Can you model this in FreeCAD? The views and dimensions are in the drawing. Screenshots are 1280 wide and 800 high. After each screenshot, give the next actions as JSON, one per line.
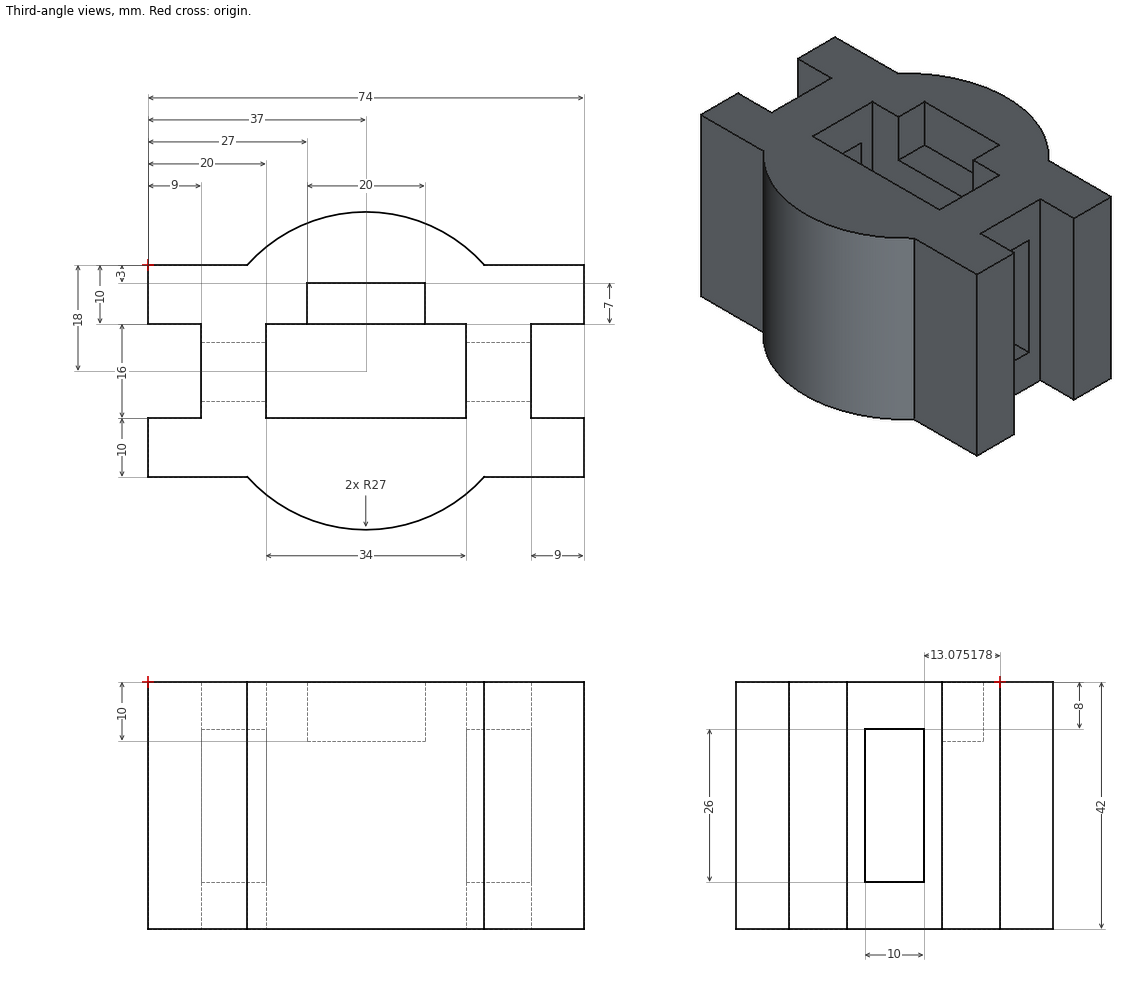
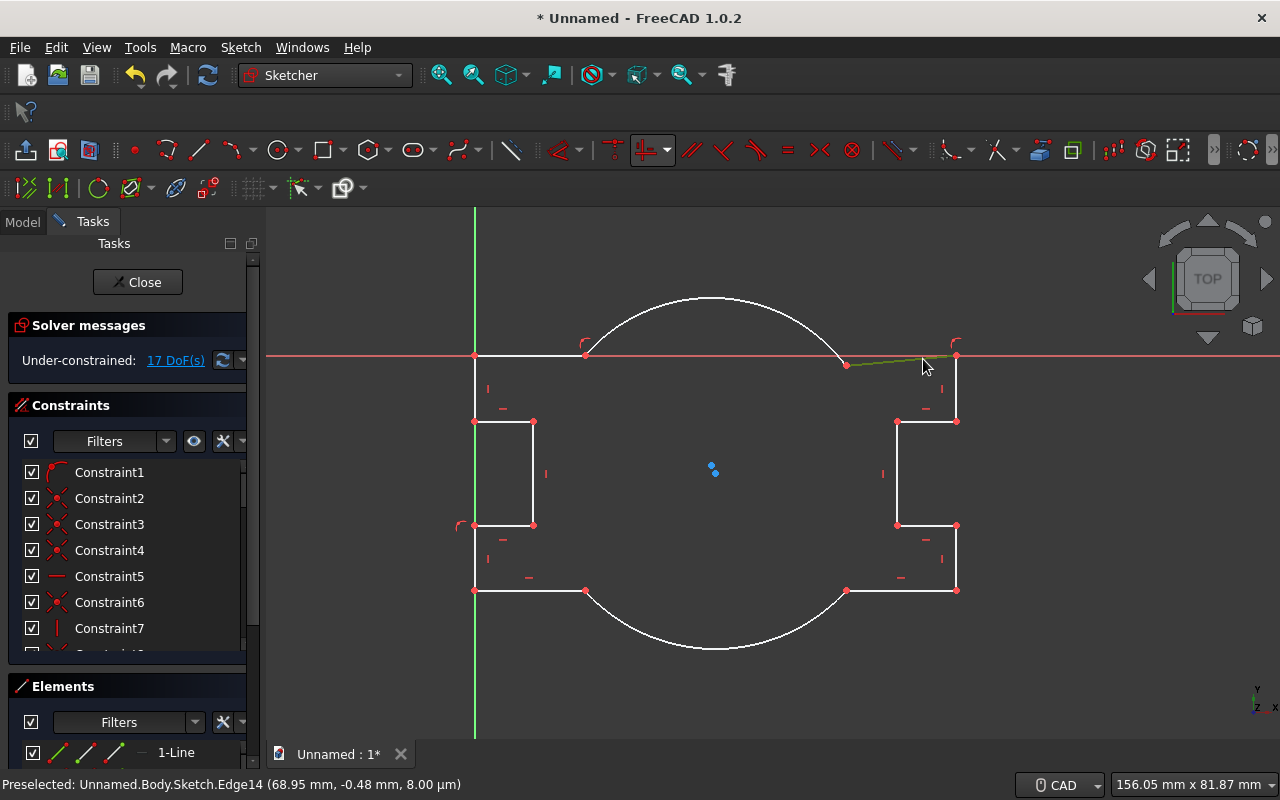
{"action": "left_click", "coordinate": [670, 150]}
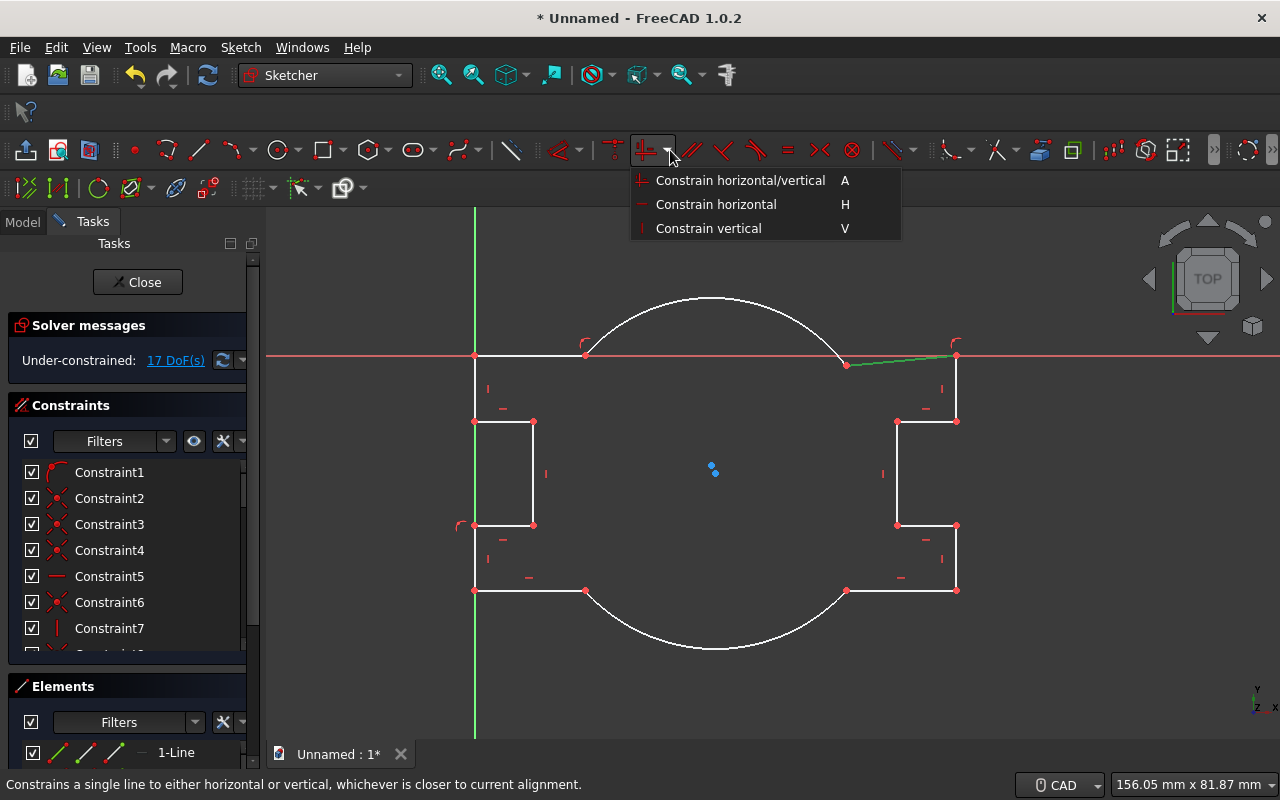
{"action": "left_click", "coordinate": [766, 204]}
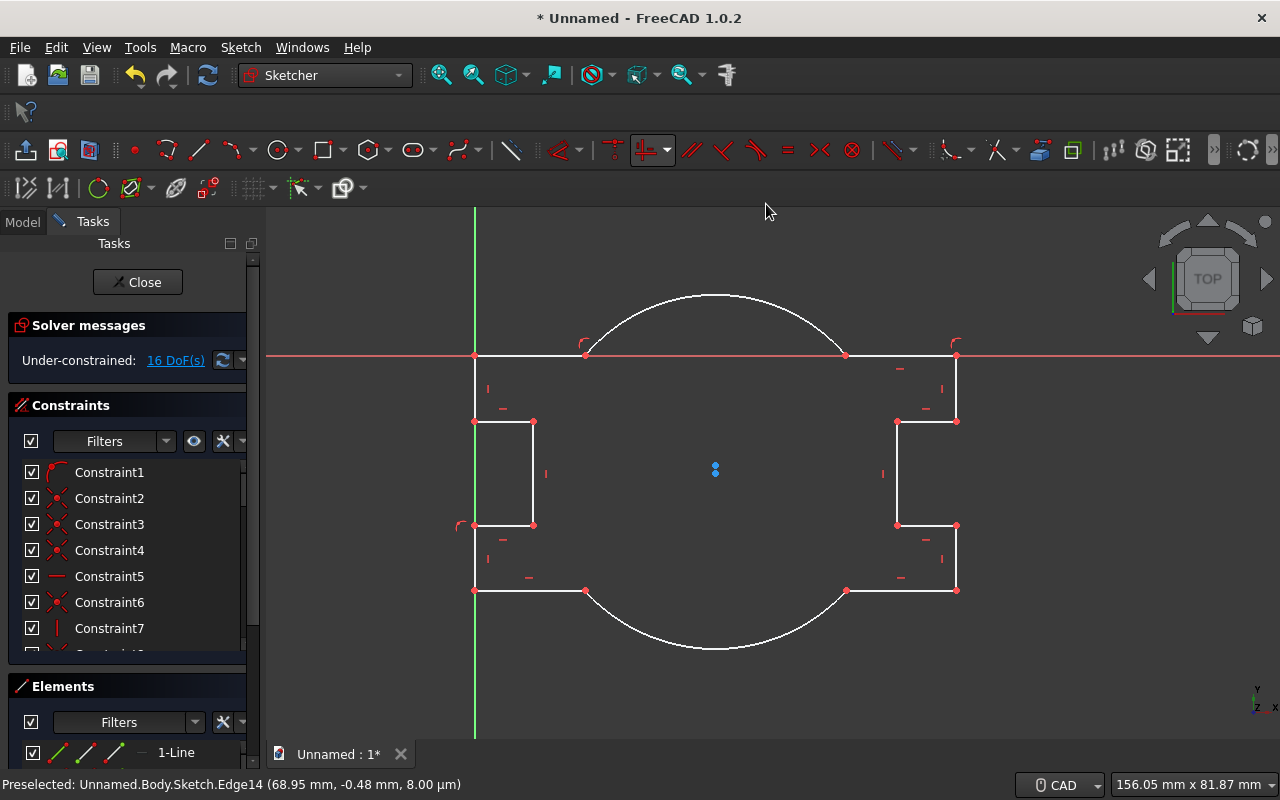
{"action": "left_click", "coordinate": [658, 639]}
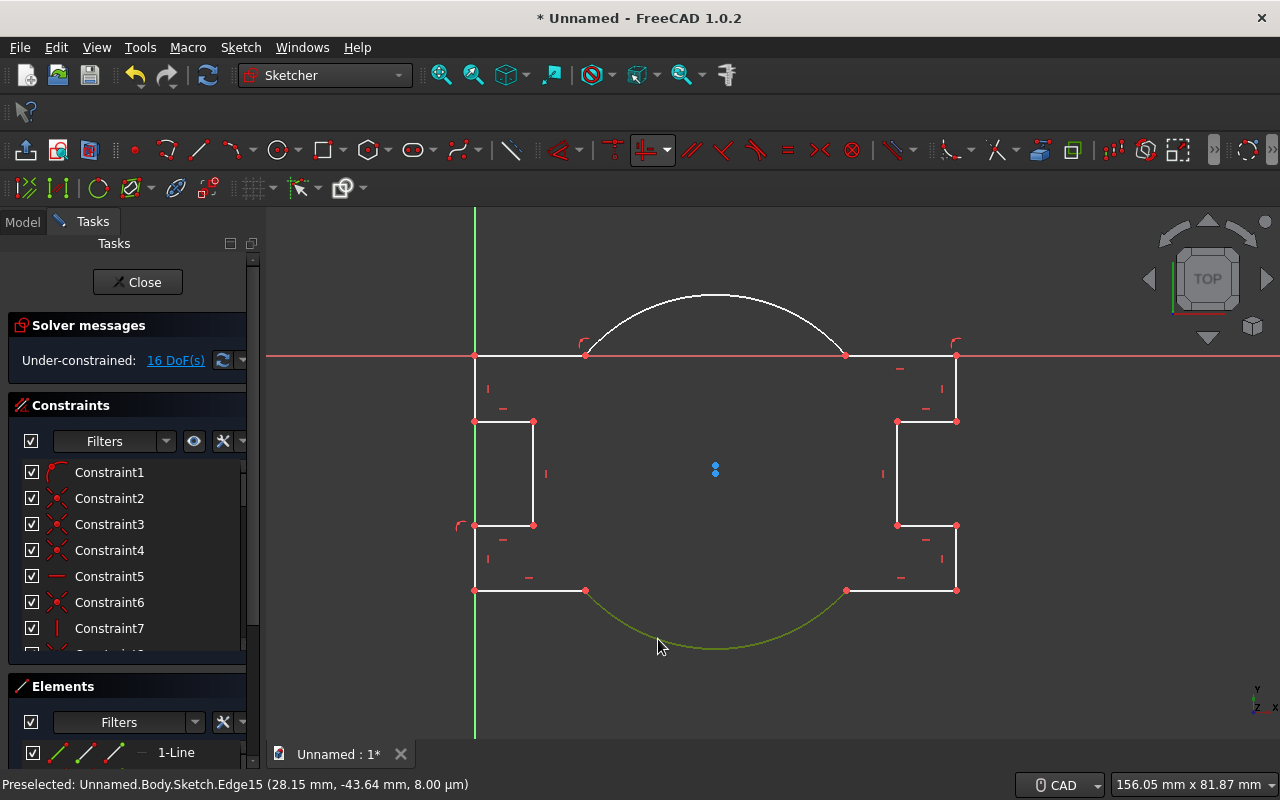
{"action": "left_click", "coordinate": [774, 305]}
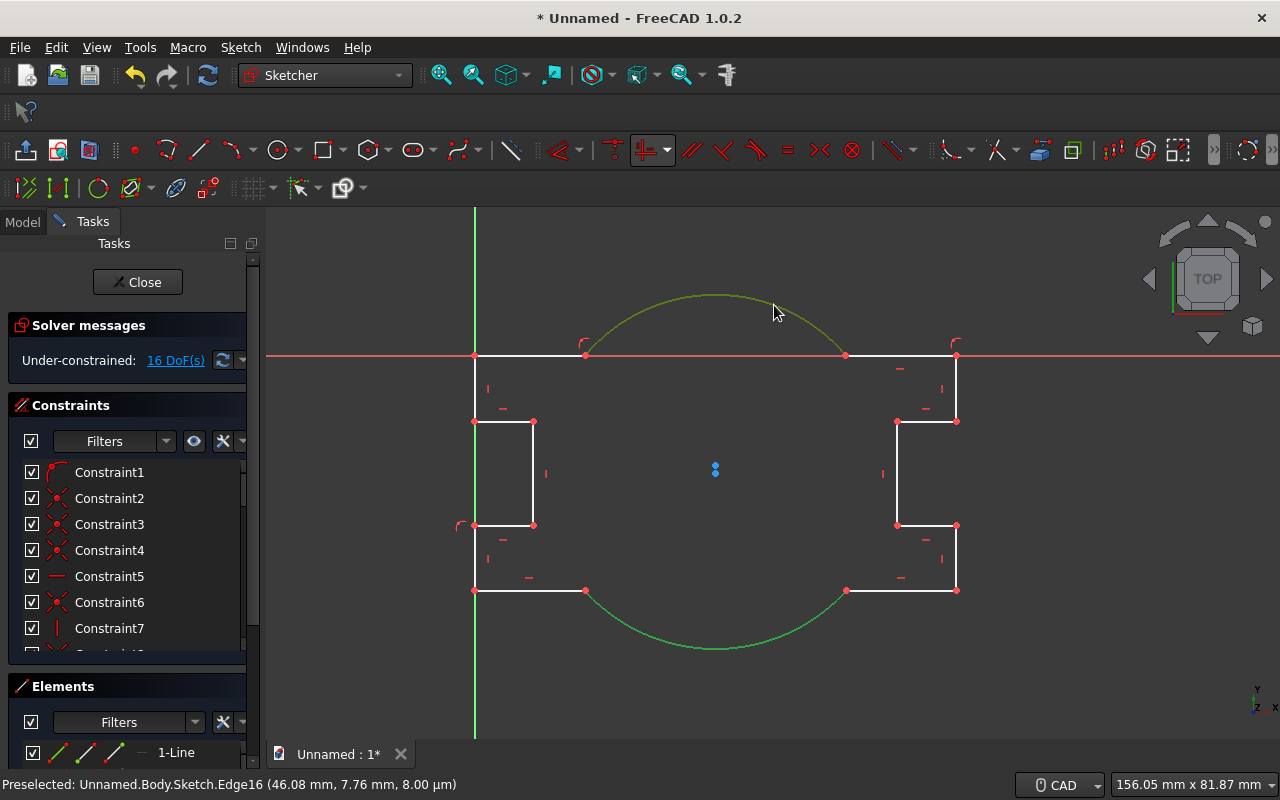
{"action": "left_click", "coordinate": [614, 150]}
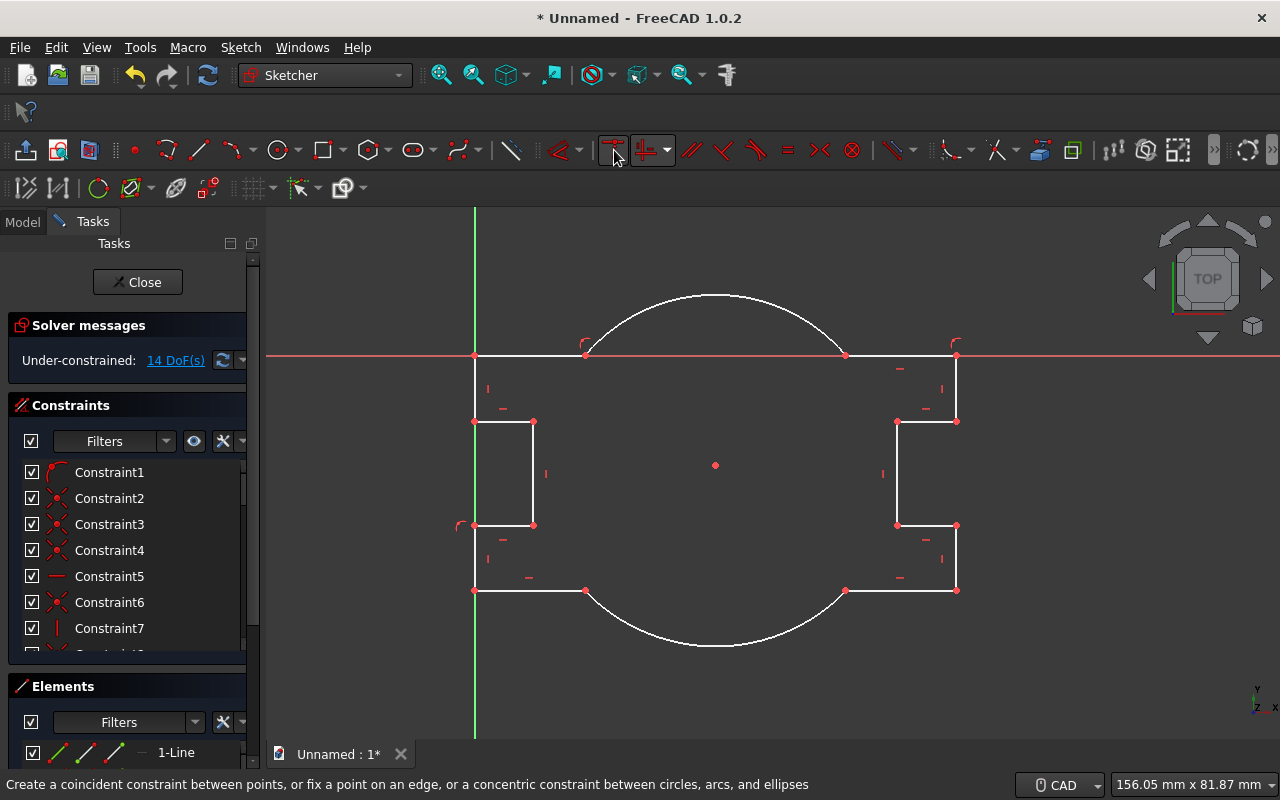
{"action": "left_click", "coordinate": [658, 637]}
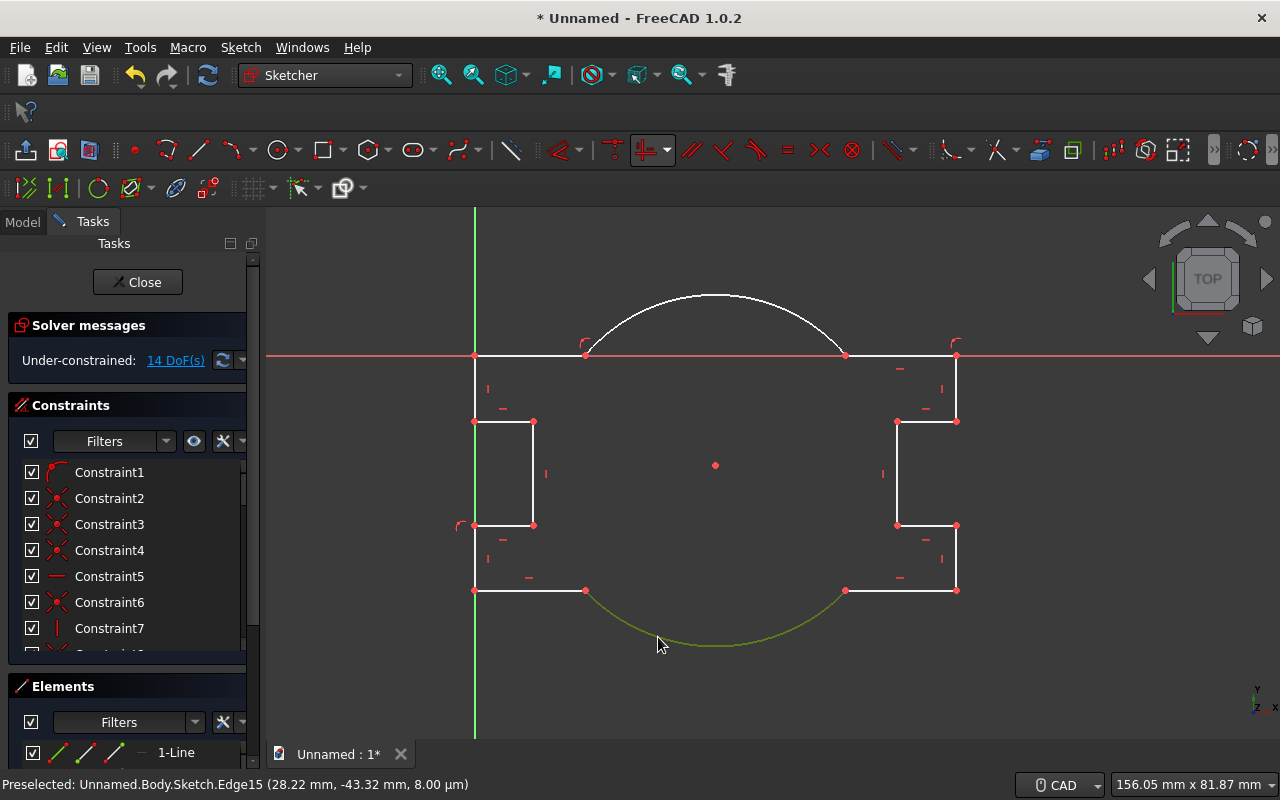
{"action": "left_click", "coordinate": [774, 305]}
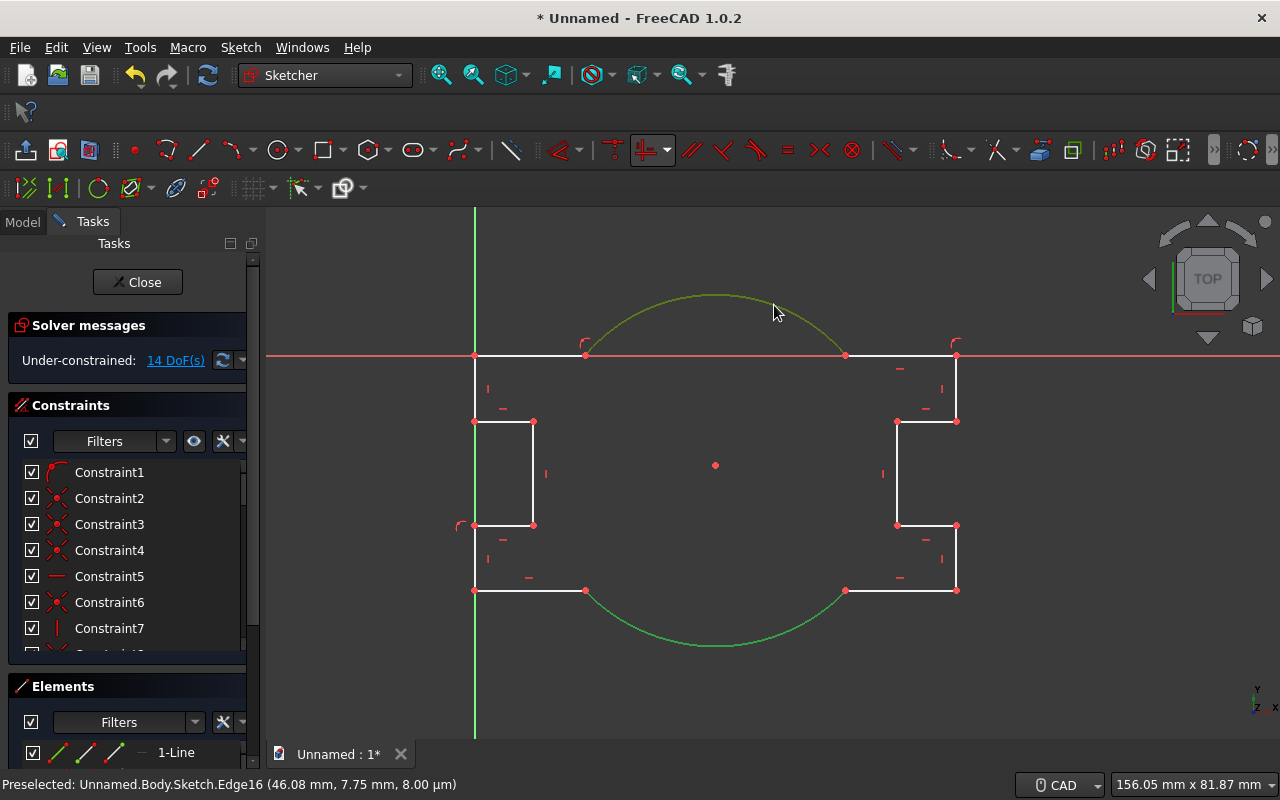
{"action": "left_click", "coordinate": [788, 150]}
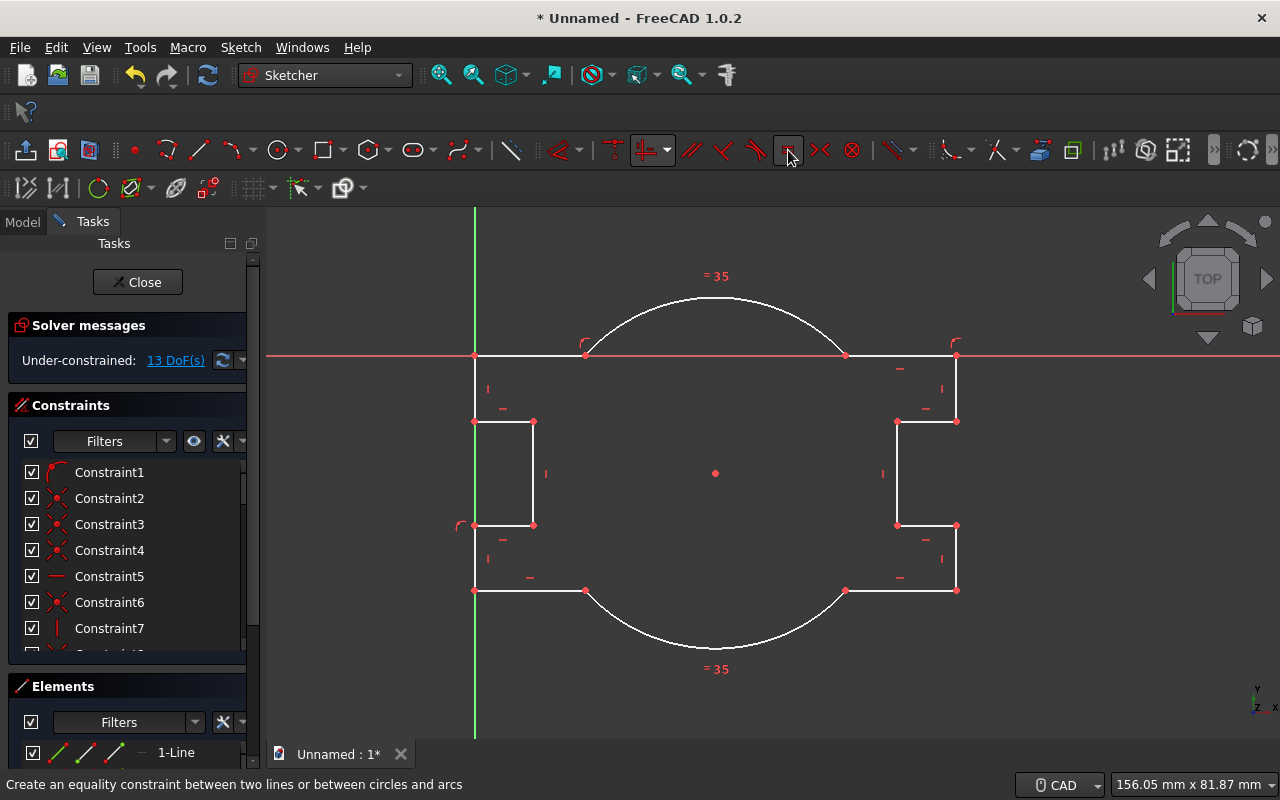
{"action": "left_click", "coordinate": [558, 150]}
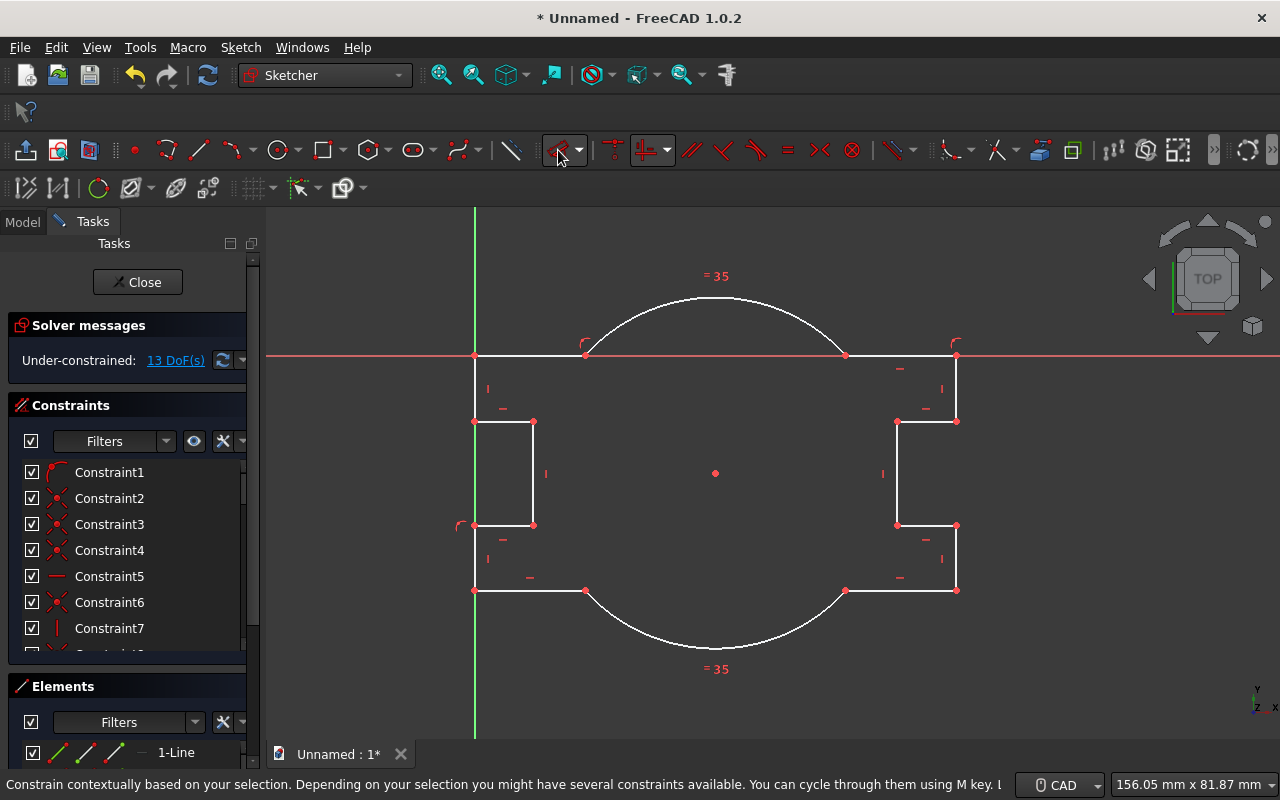
{"action": "left_click", "coordinate": [658, 639]}
{"action": "left_click", "coordinate": [648, 669]}